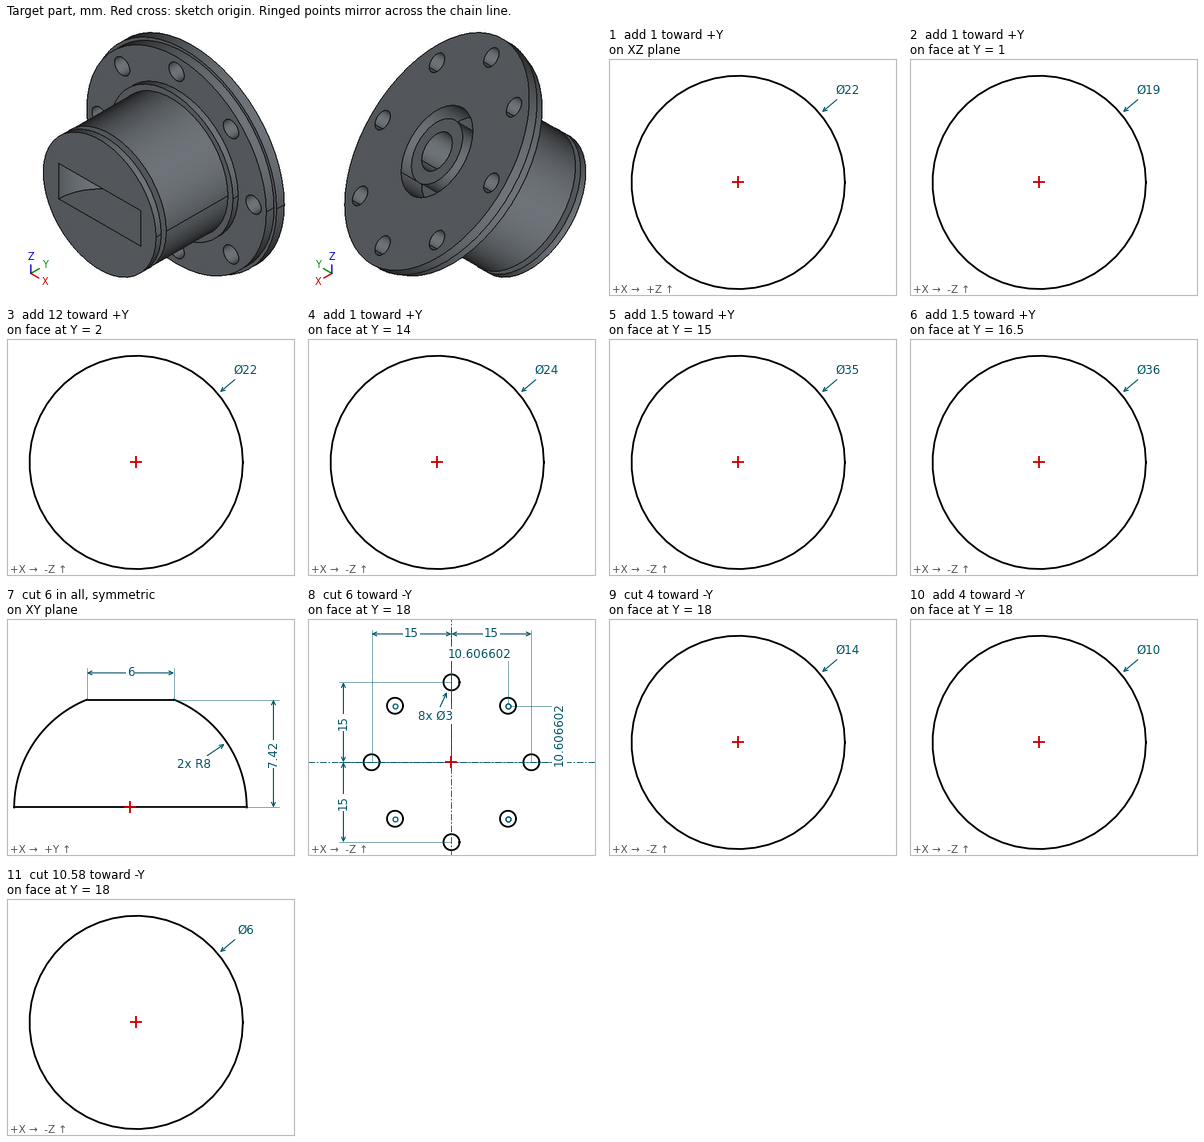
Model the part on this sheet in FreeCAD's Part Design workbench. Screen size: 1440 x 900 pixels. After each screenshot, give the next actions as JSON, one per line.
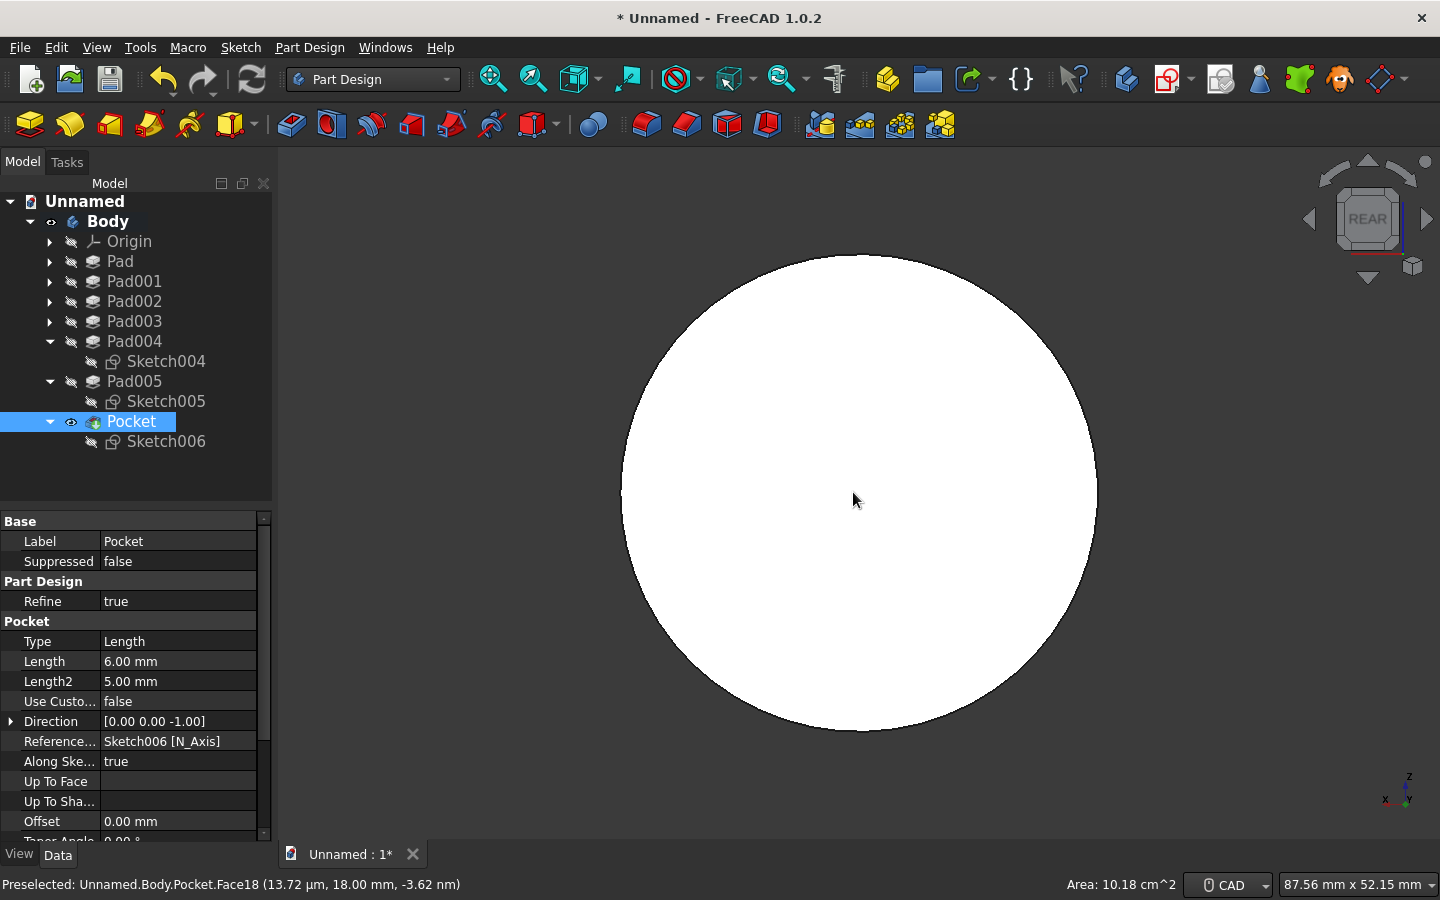
{"action": "left_click", "coordinate": [1168, 80]}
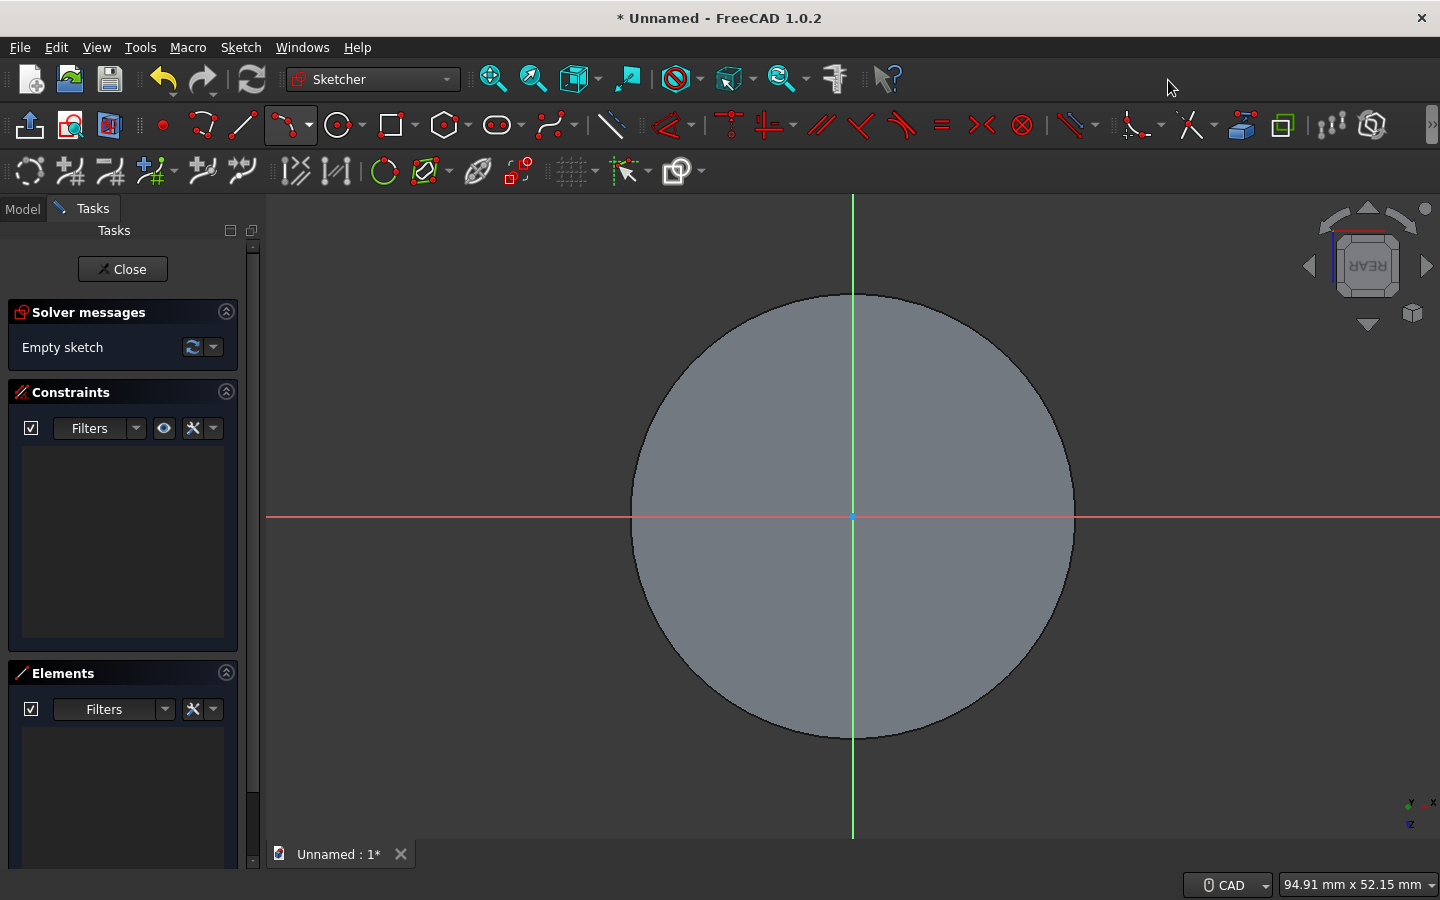
{"action": "left_click", "coordinate": [338, 126]}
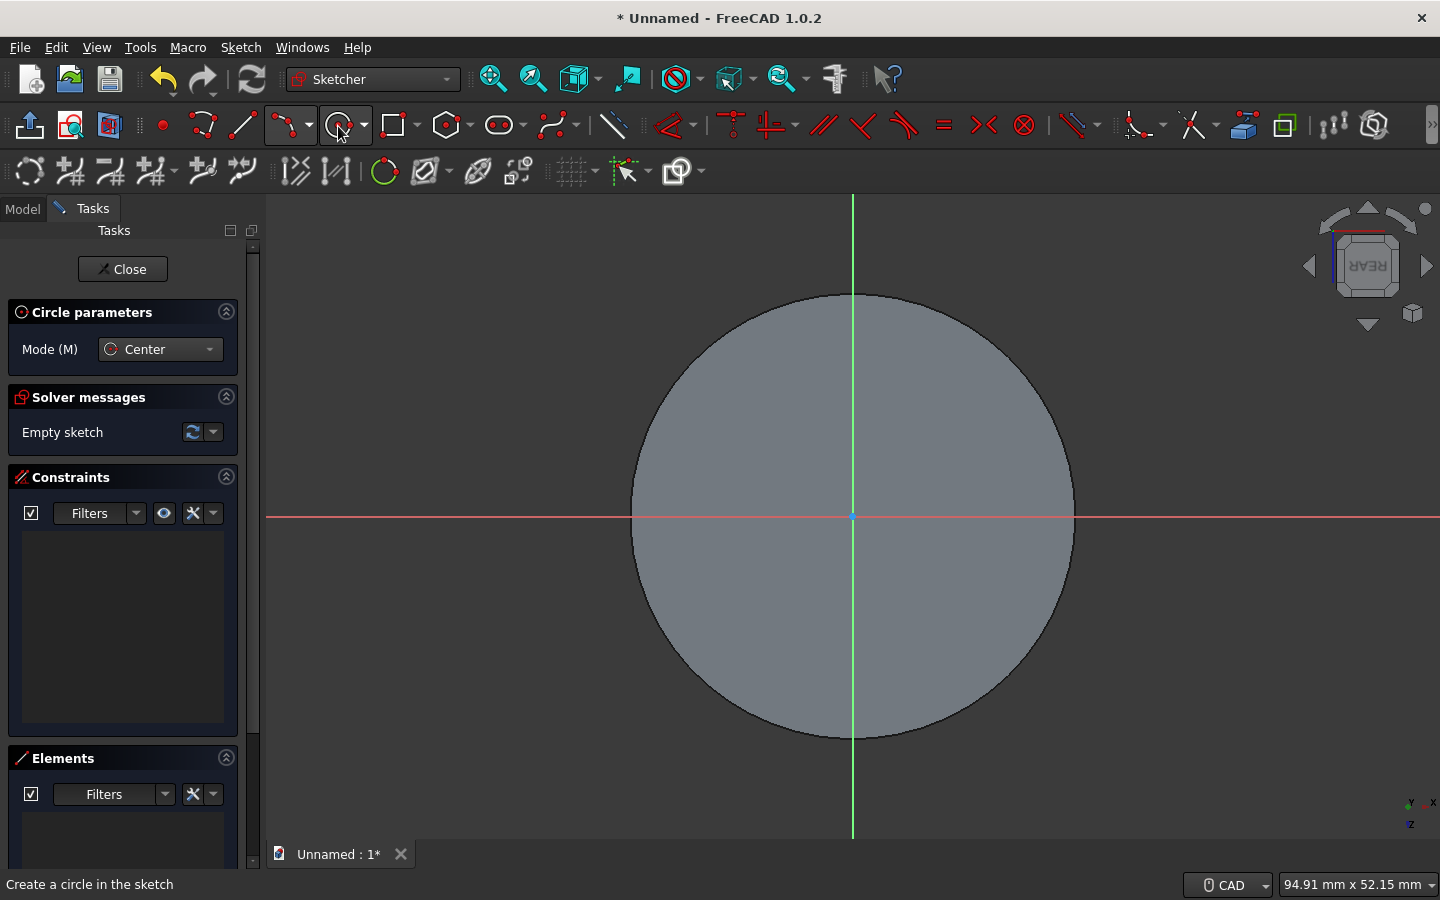
{"action": "scroll", "coordinate": [853, 331], "scroll_direction": "up", "scroll_amount": 2}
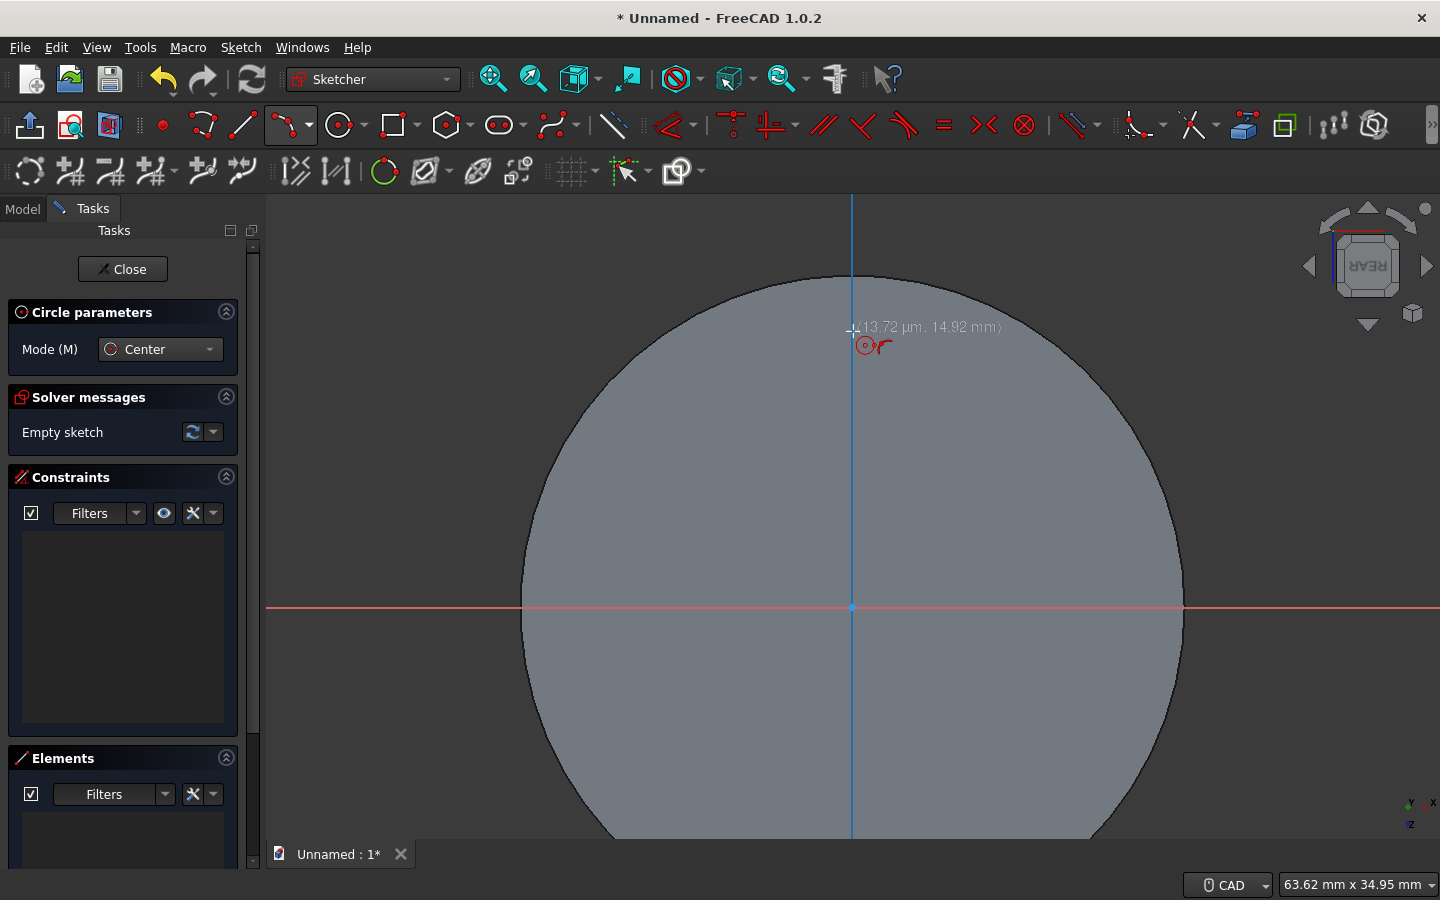
{"action": "left_click", "coordinate": [853, 331]}
{"action": "mouse_move", "coordinate": [872, 311]}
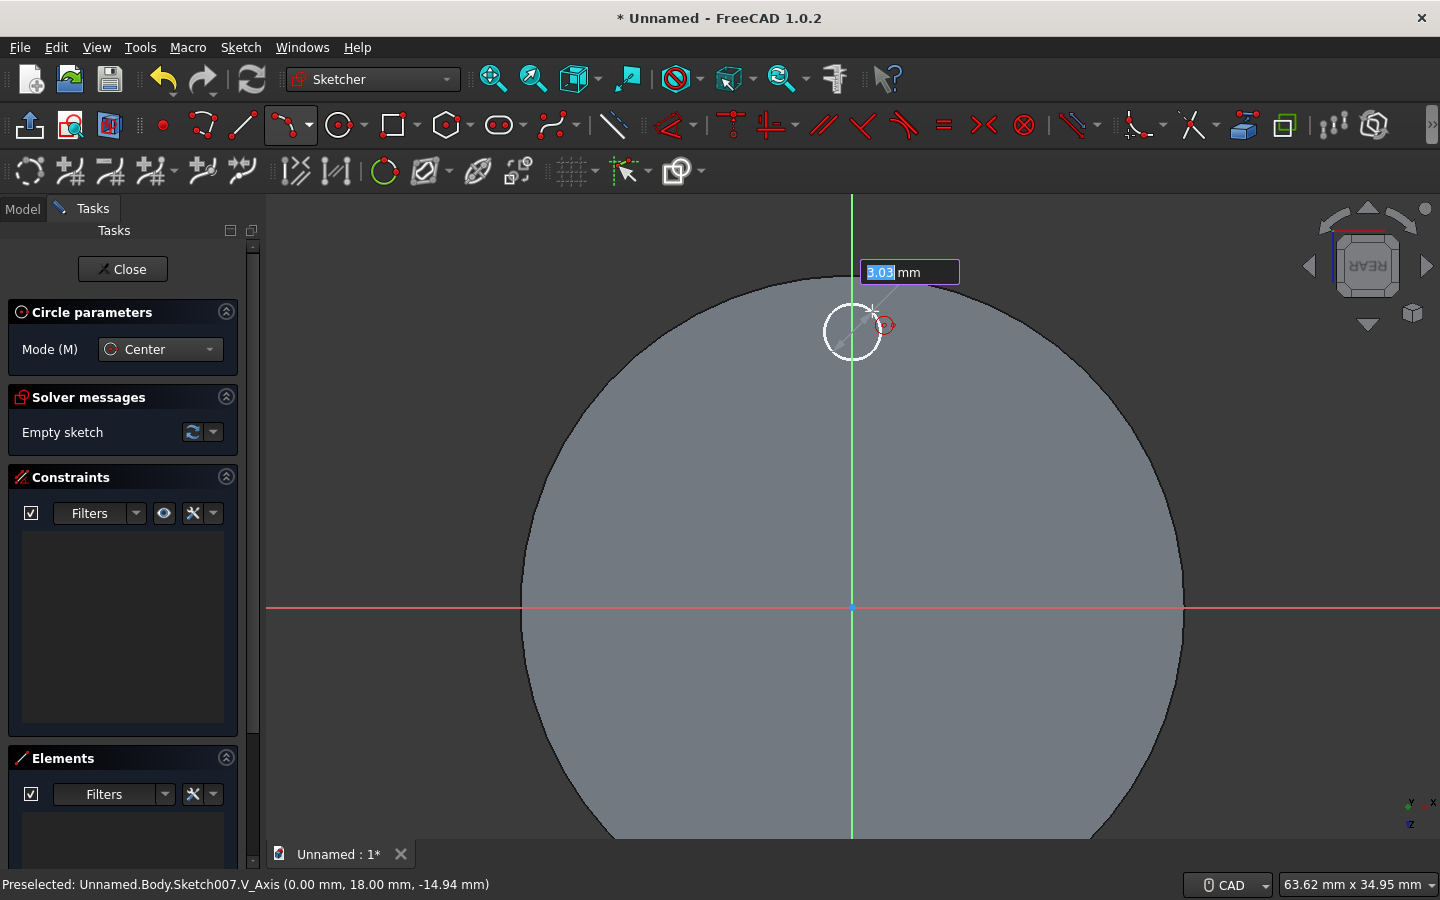
{"action": "type", "text": "3"}
{"action": "key", "text": "Return"}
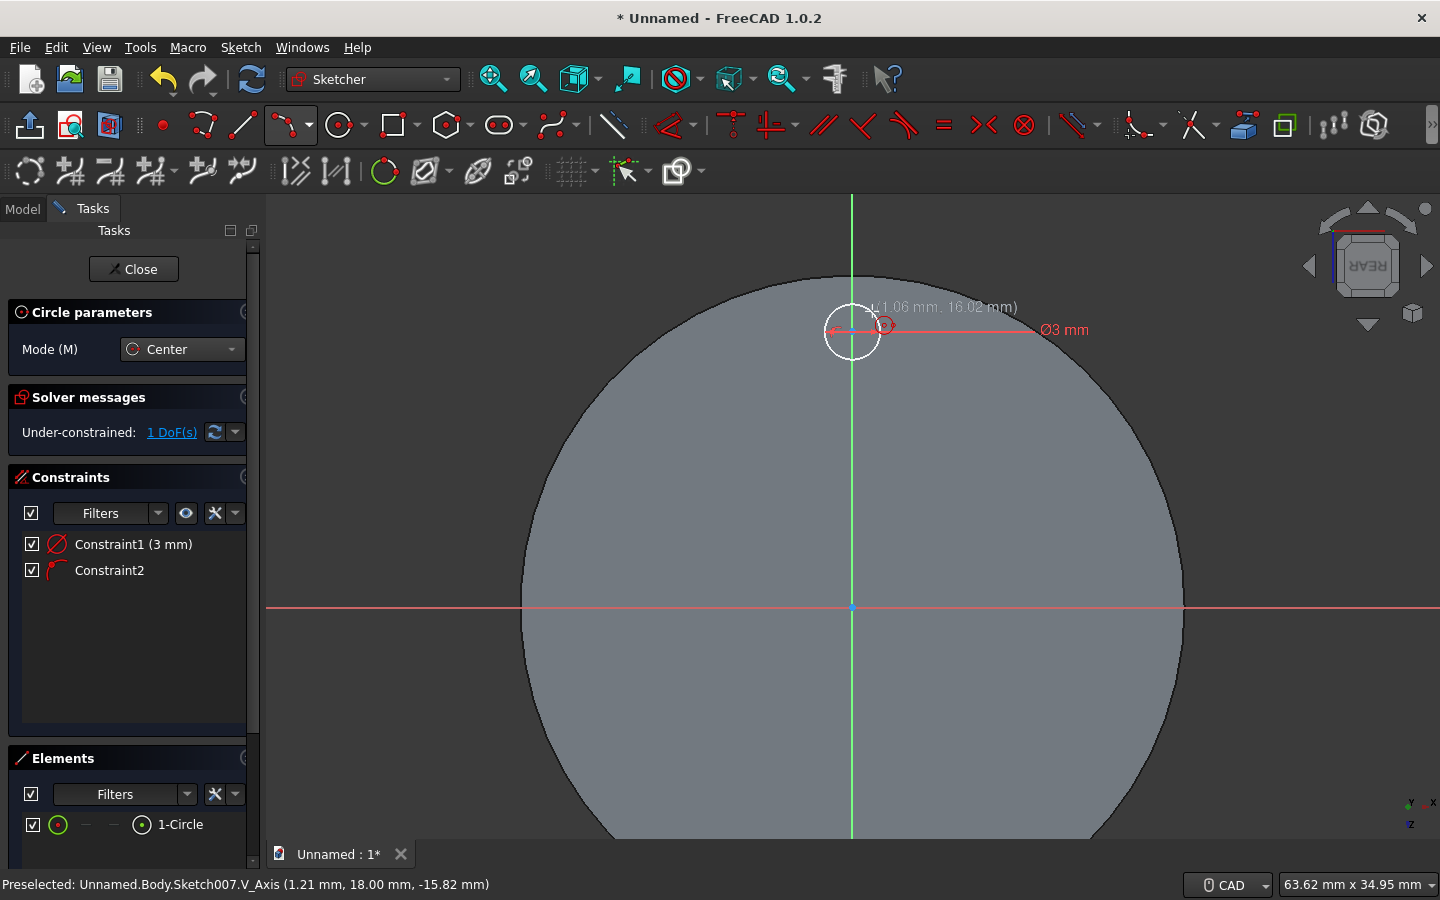
{"action": "left_click", "coordinate": [1048, 412]}
{"action": "mouse_move", "coordinate": [1068, 392]}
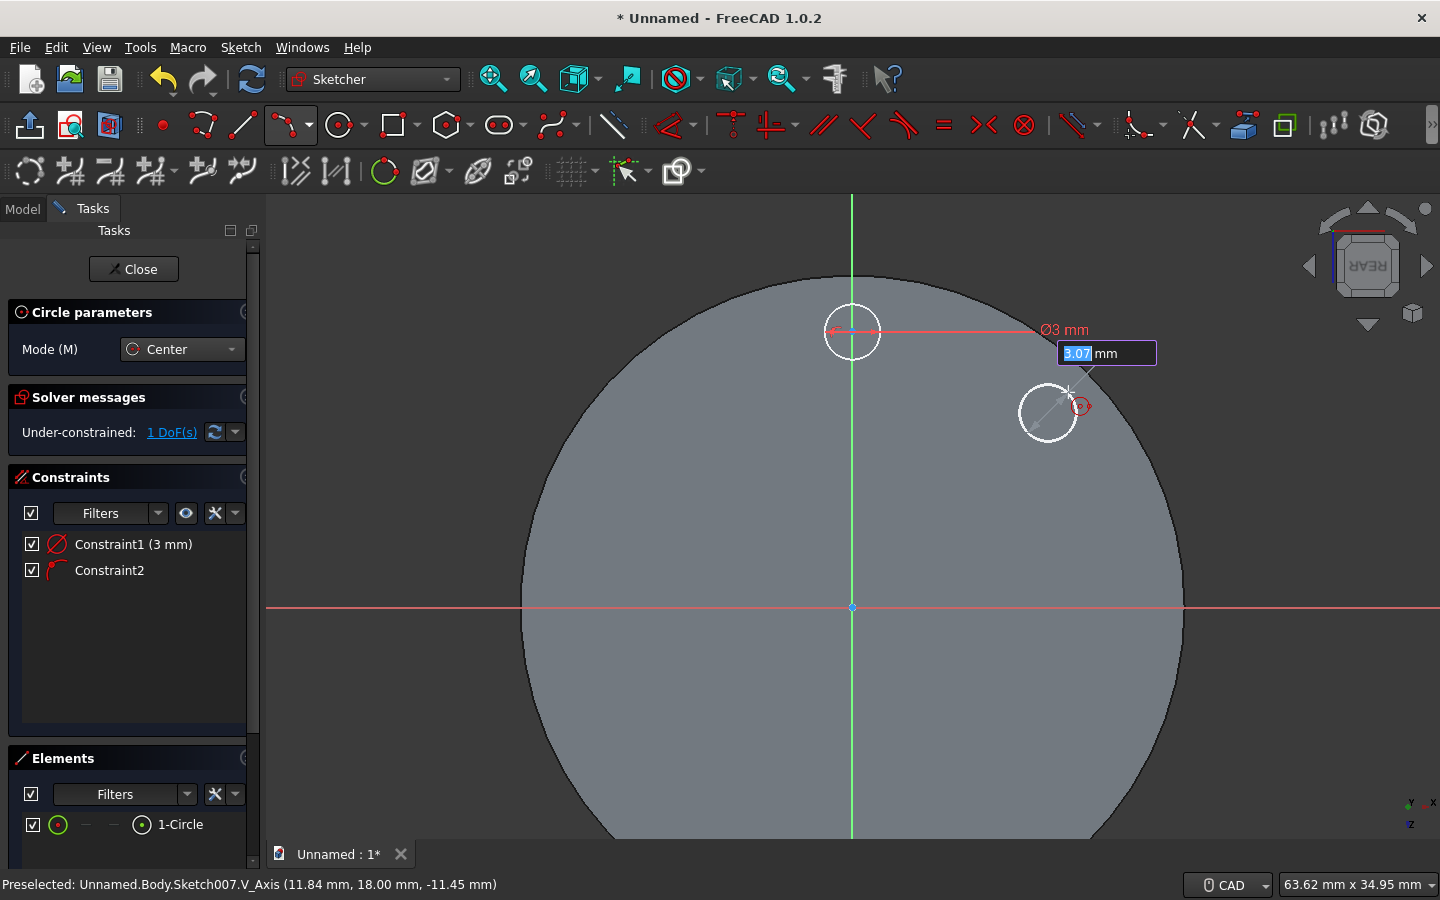
{"action": "type", "text": "3"}
{"action": "key", "text": "Return"}